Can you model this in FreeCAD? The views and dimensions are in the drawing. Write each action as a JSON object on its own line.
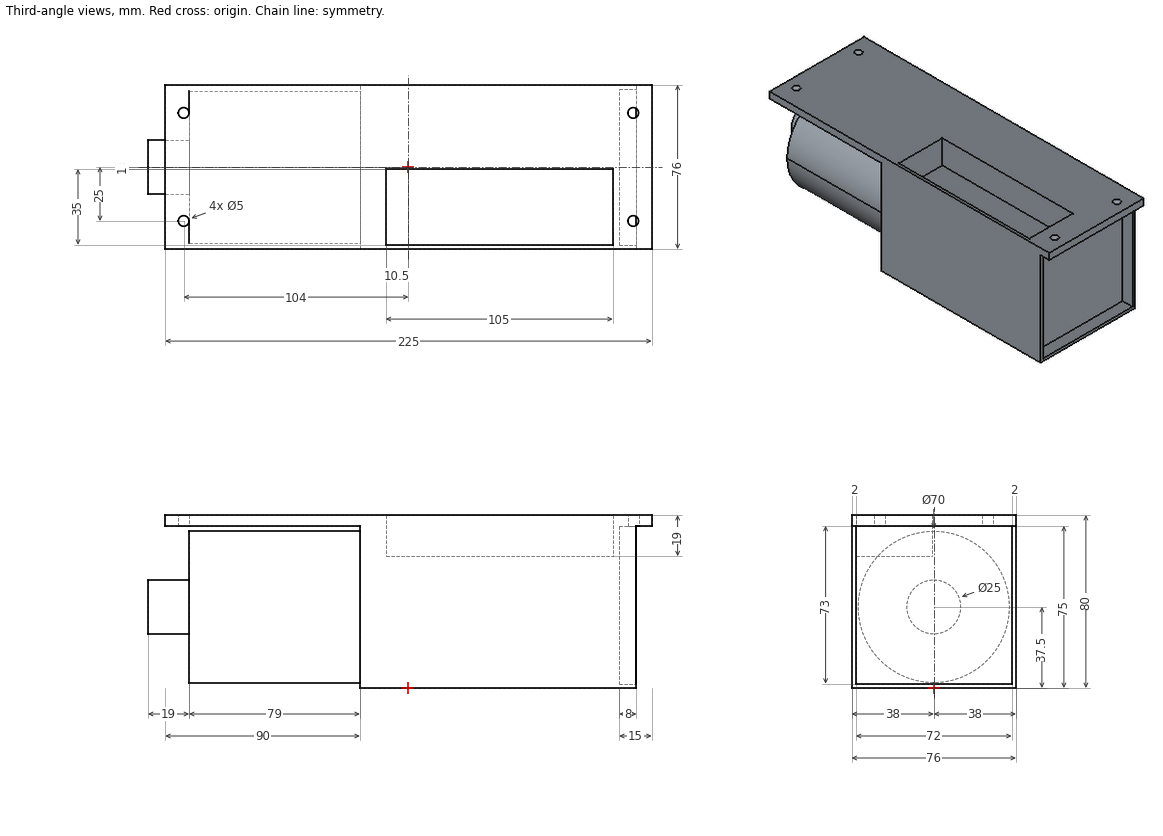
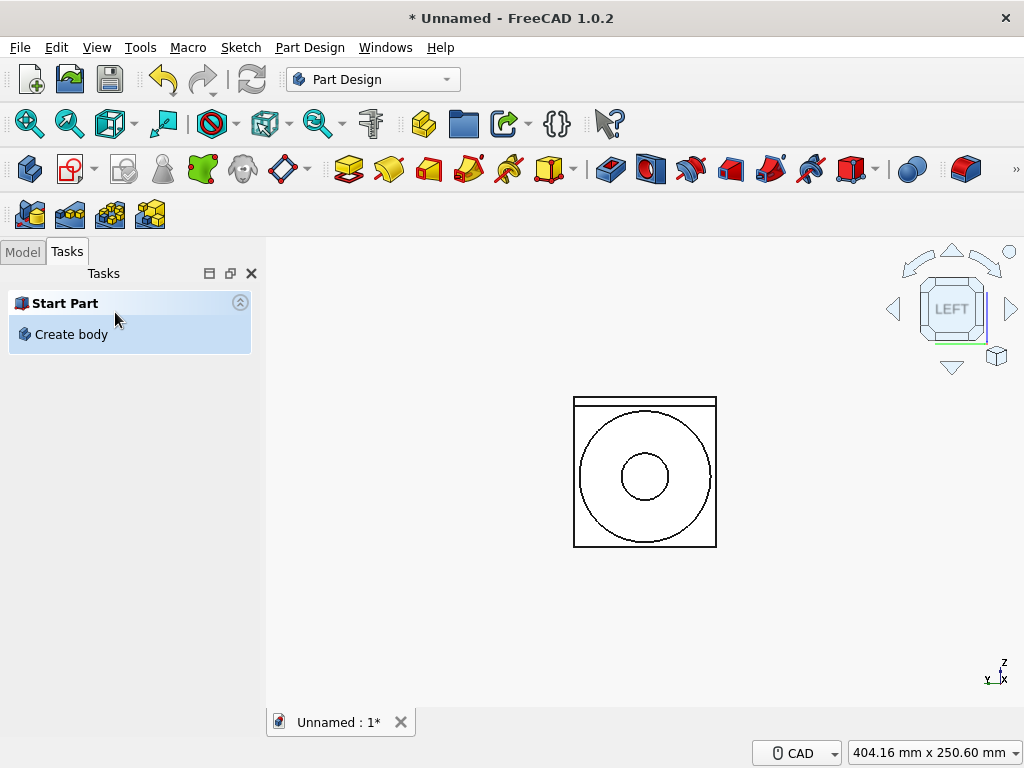
{"action": "key", "text": "v f"}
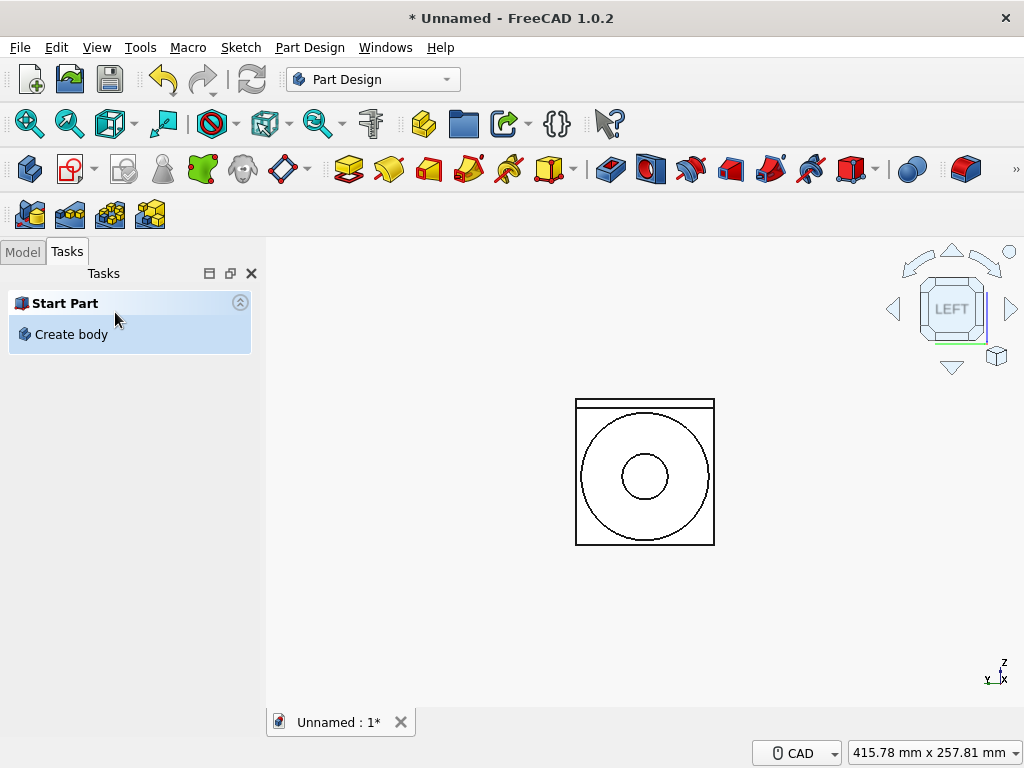
{"action": "key", "text": "0"}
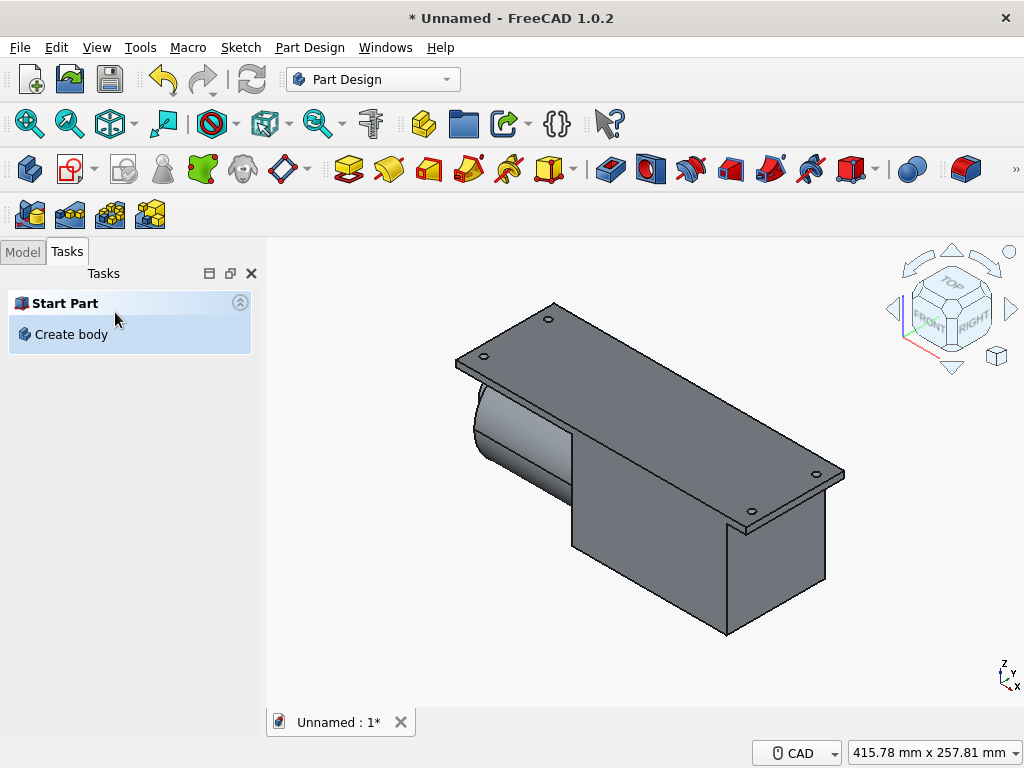
{"action": "left_click", "coordinate": [733, 462]}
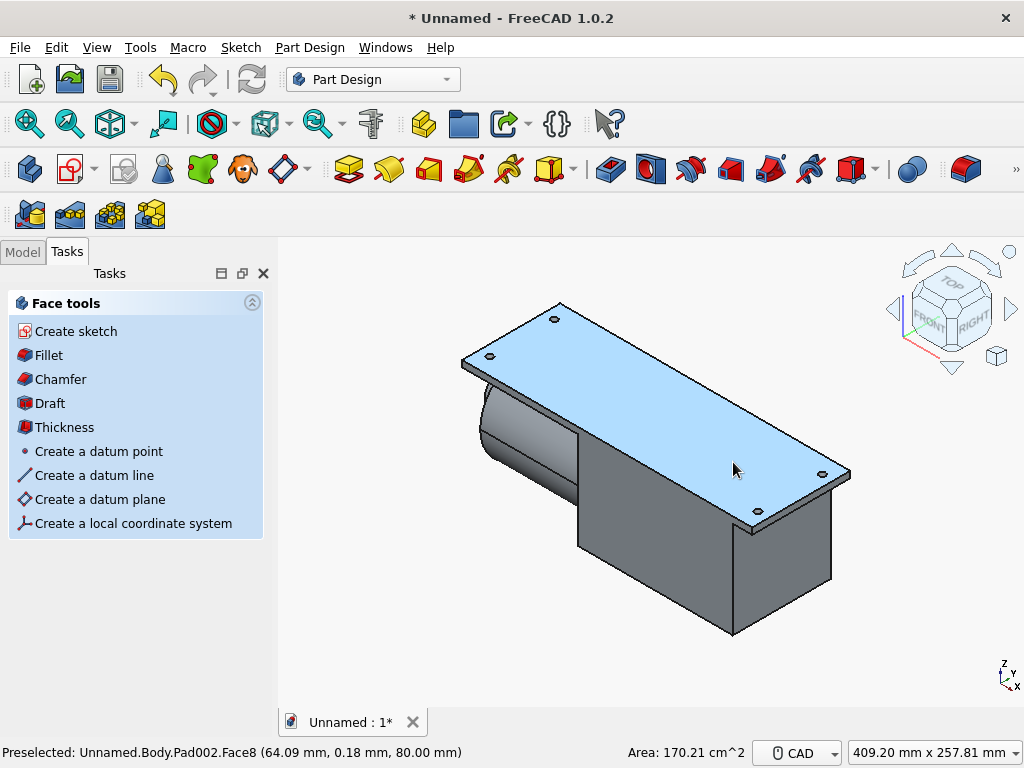
{"action": "left_click", "coordinate": [70, 170]}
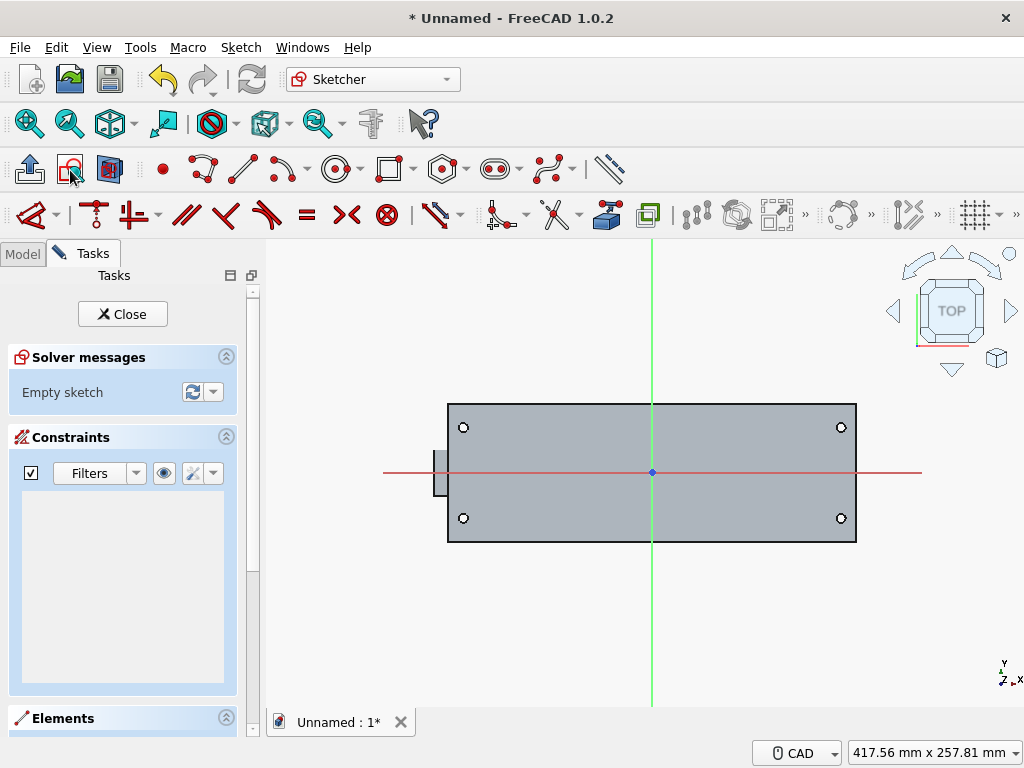
{"action": "scroll", "coordinate": [853, 532], "scroll_direction": "up", "scroll_amount": 4}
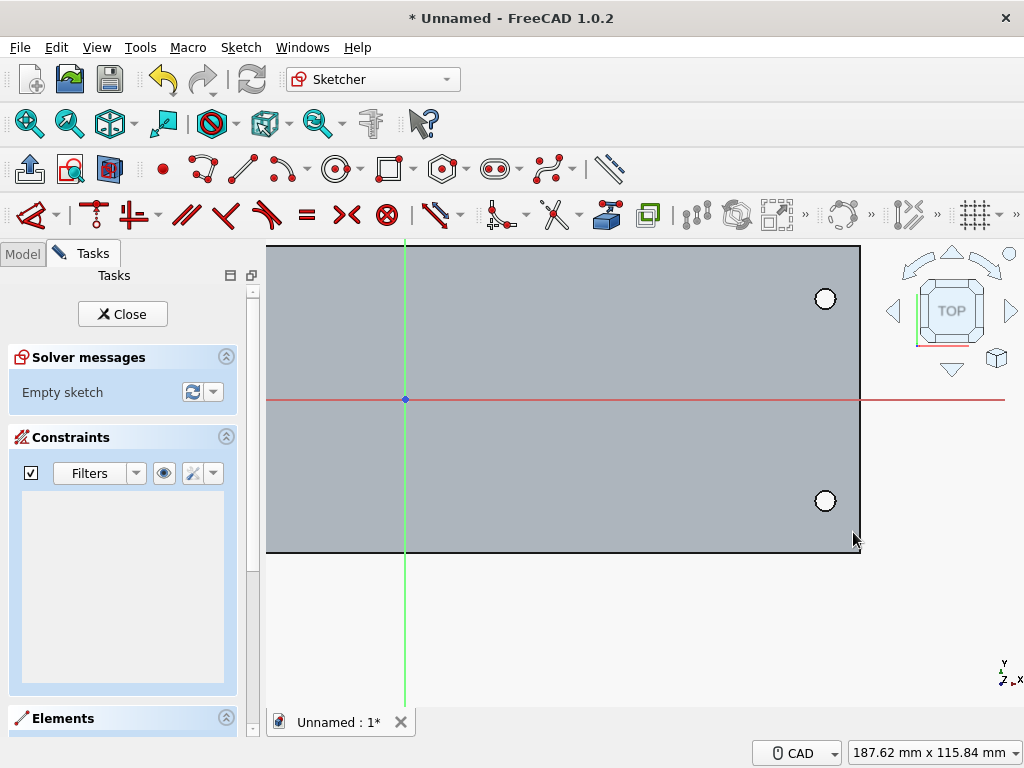
{"action": "key", "text": "g r"}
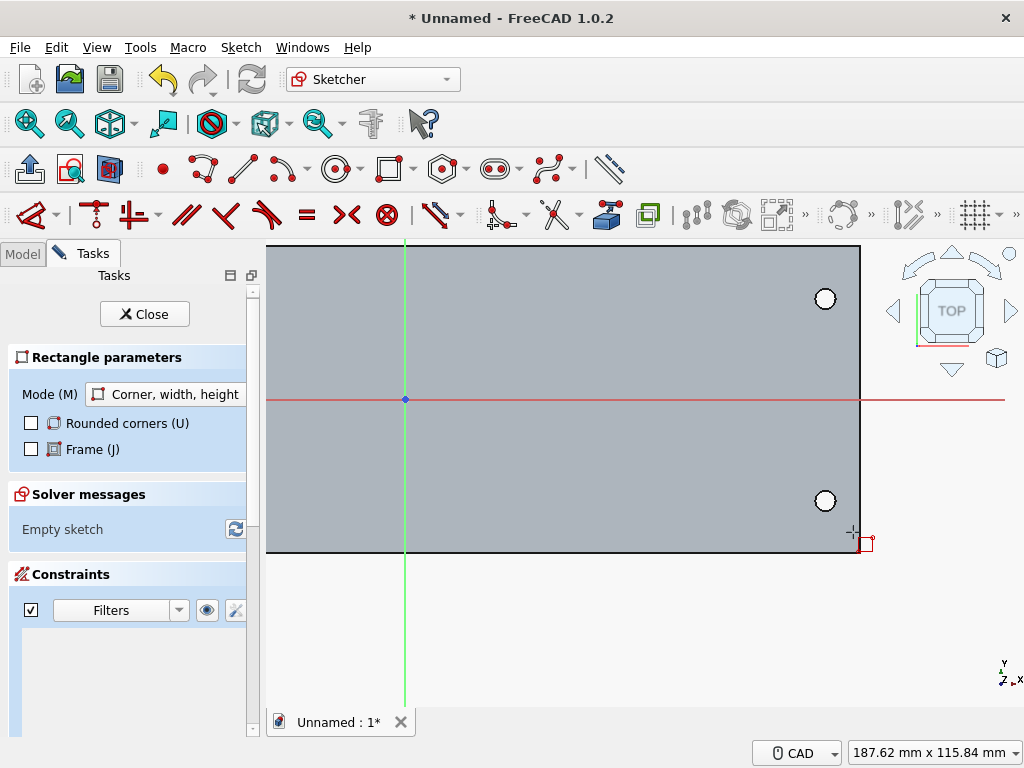
{"action": "scroll", "coordinate": [363, 404], "scroll_direction": "up", "scroll_amount": 7}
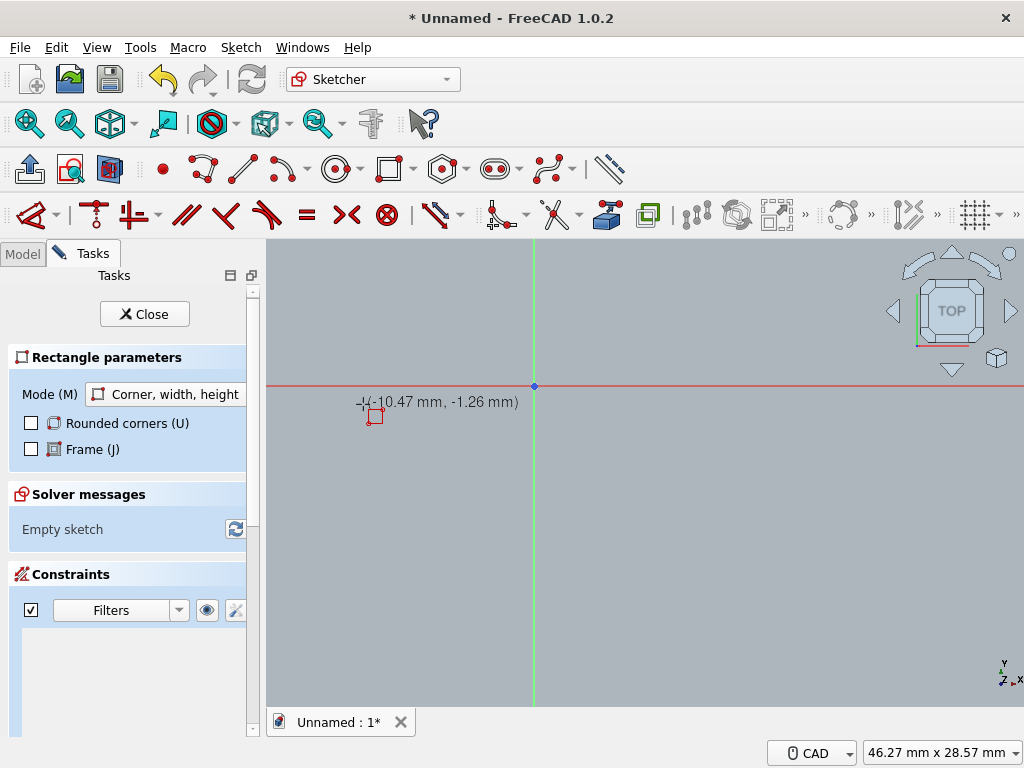
{"action": "left_click", "coordinate": [362, 403]}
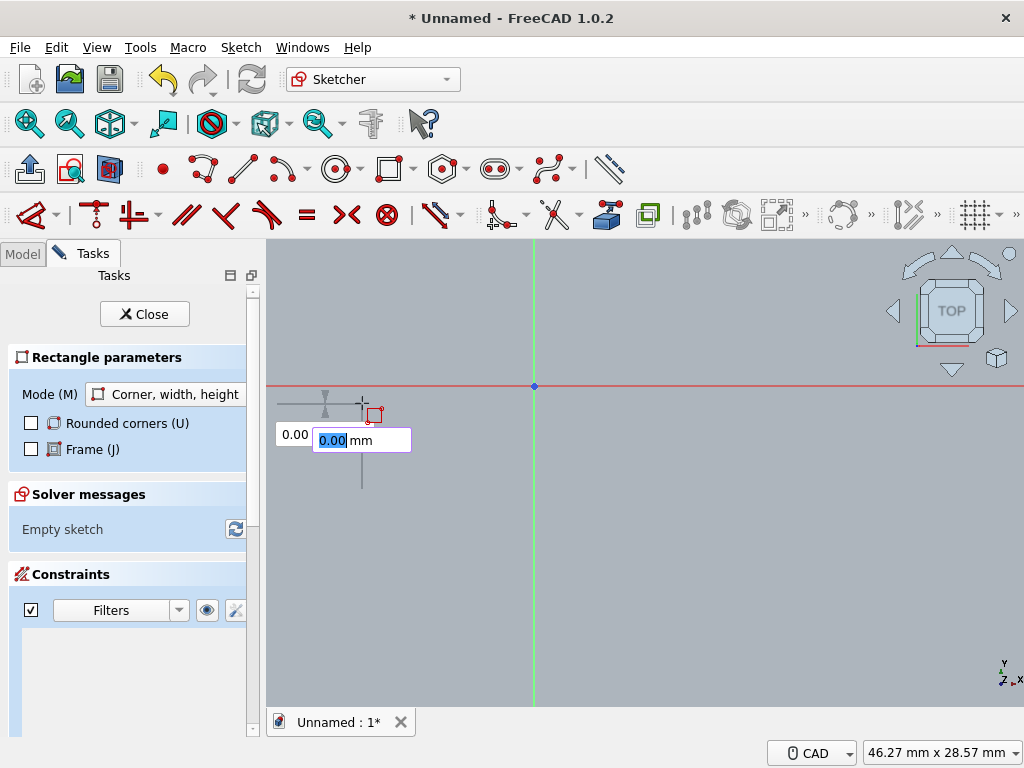
{"action": "scroll", "coordinate": [365, 405], "scroll_direction": "down", "scroll_amount": 7}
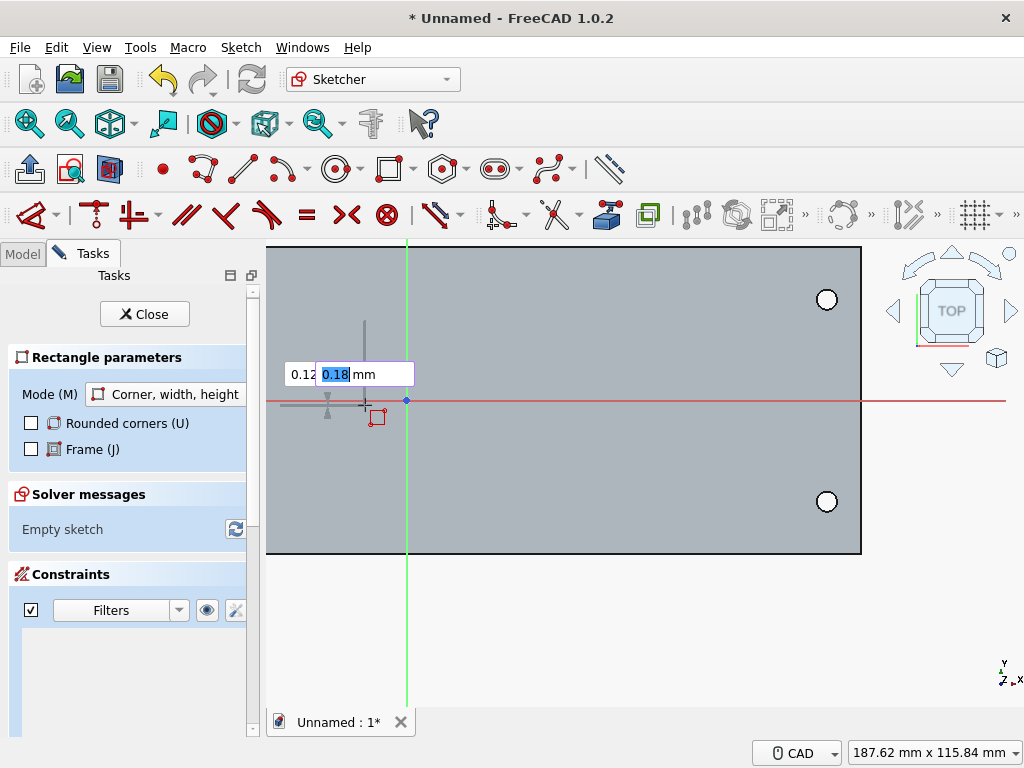
{"action": "left_click", "coordinate": [789, 546]}
{"action": "key", "text": "Escape"}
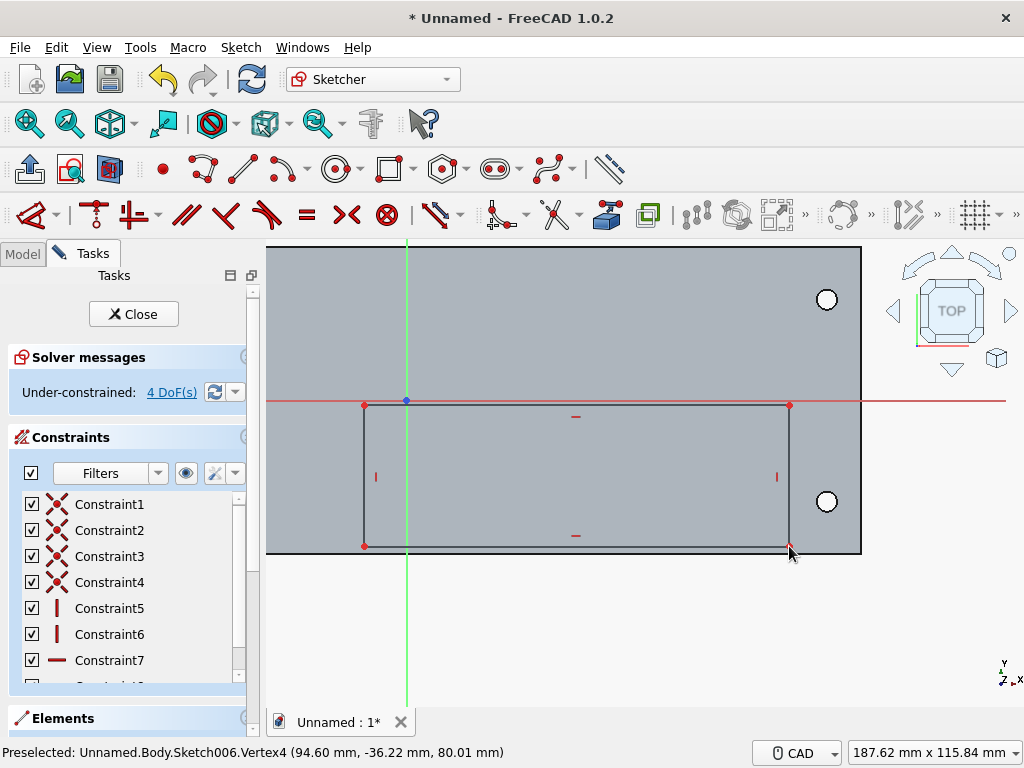
{"action": "key", "text": "d"}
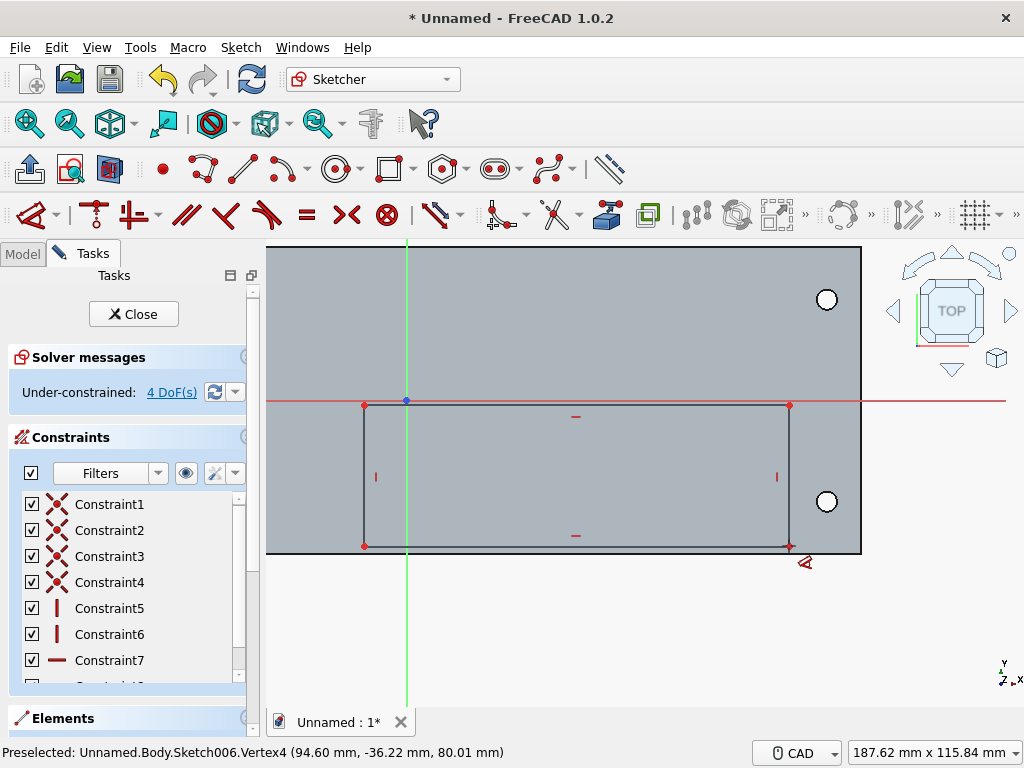
{"action": "left_click", "coordinate": [364, 448]}
{"action": "left_click", "coordinate": [330, 476]}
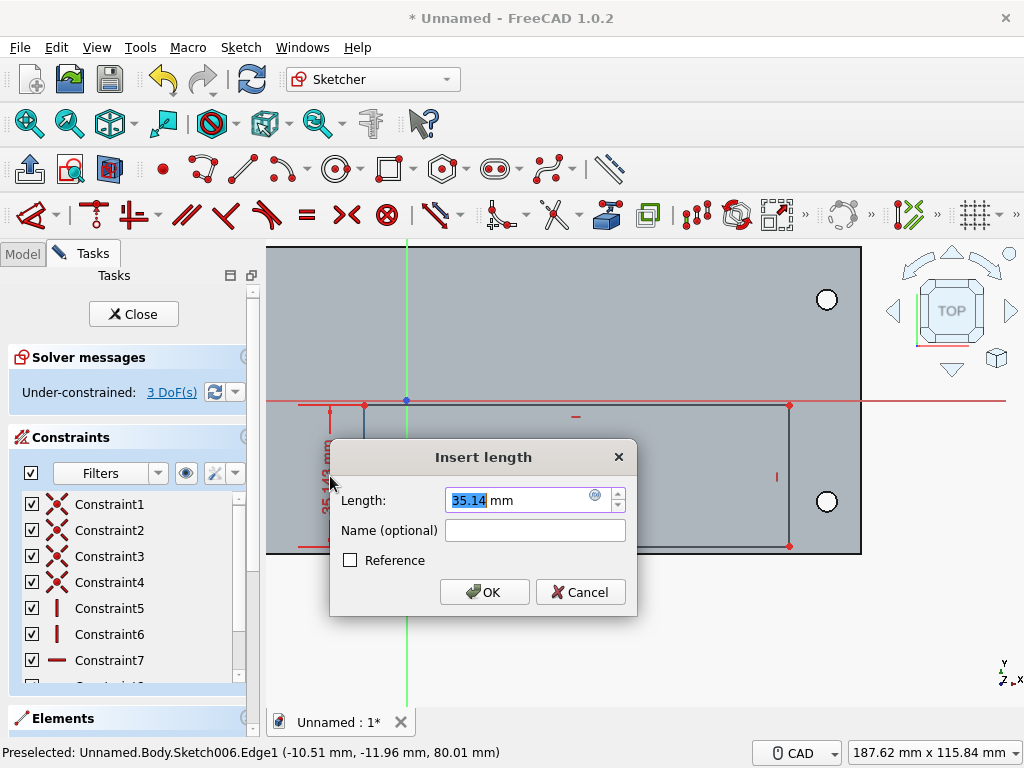
{"action": "type", "text": "35"}
{"action": "key", "text": "Return"}